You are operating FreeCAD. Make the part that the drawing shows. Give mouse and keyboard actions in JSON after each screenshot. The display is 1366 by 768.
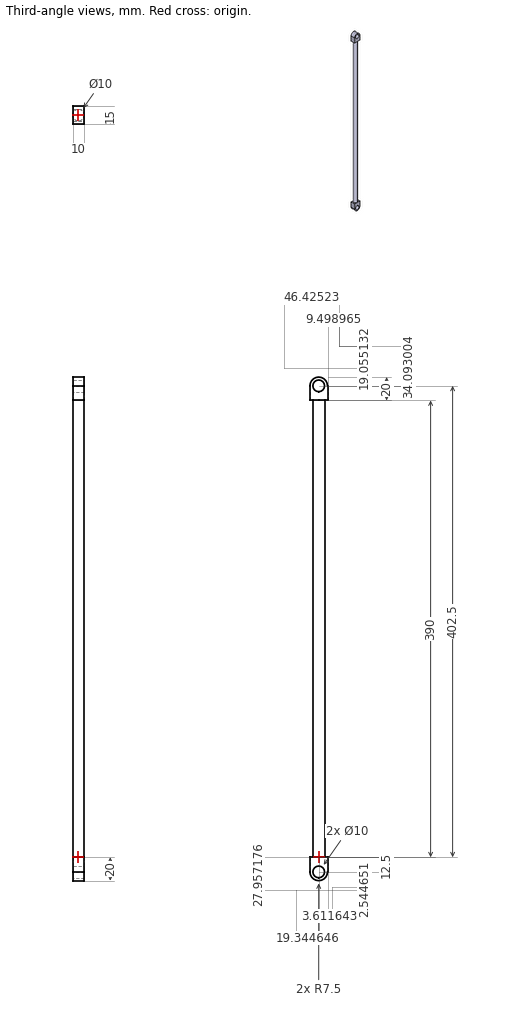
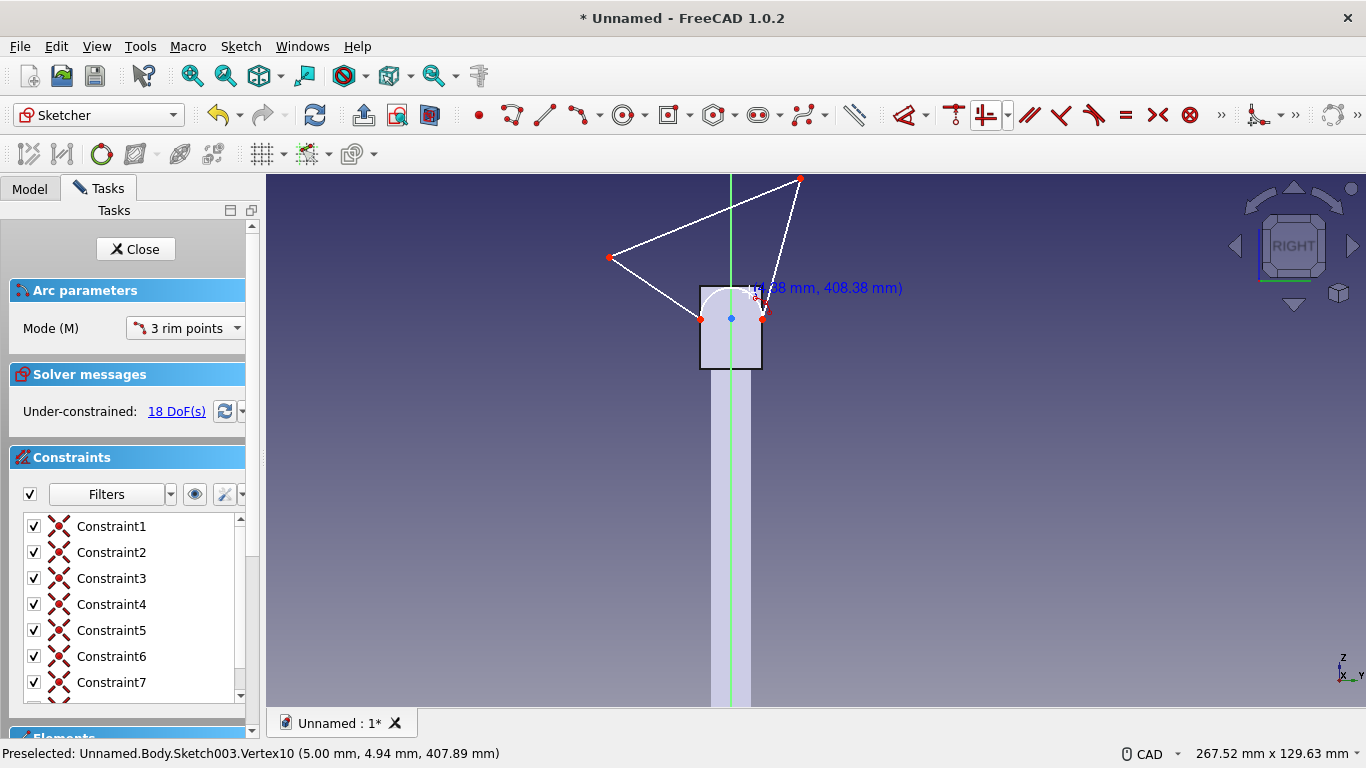
{"action": "left_click", "coordinate": [622, 116]}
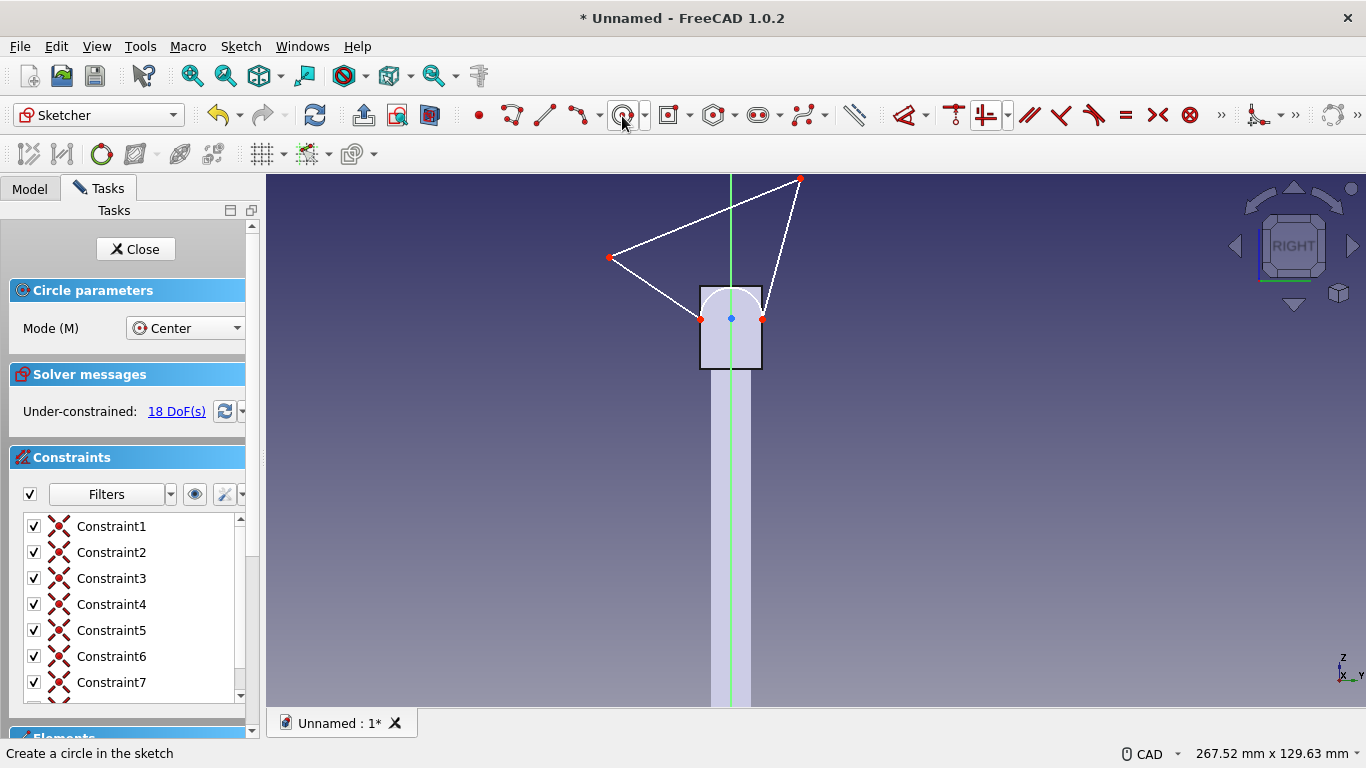
{"action": "scroll", "coordinate": [756, 304], "scroll_direction": "down", "scroll_amount": 9}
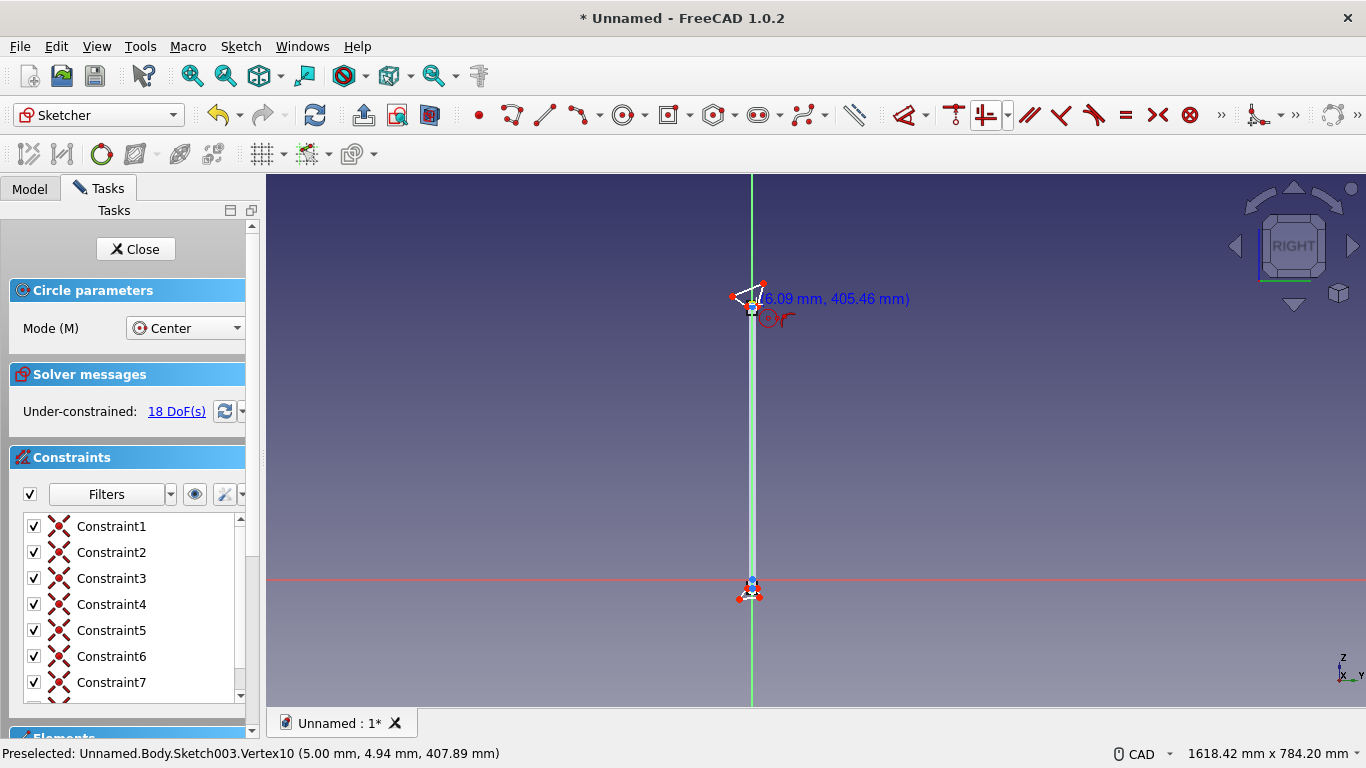
{"action": "scroll", "coordinate": [752, 588], "scroll_direction": "up", "scroll_amount": 10}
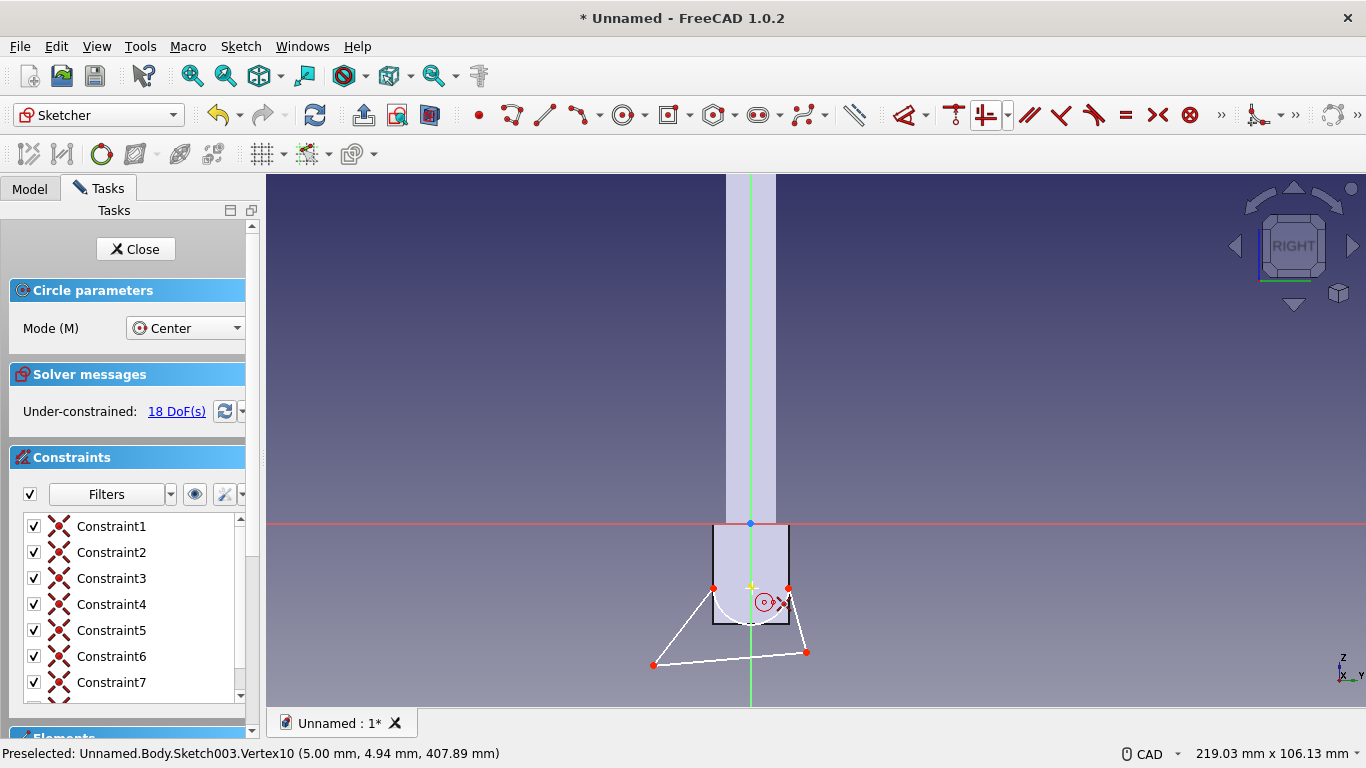
{"action": "left_click", "coordinate": [751, 586]}
{"action": "mouse_move", "coordinate": [769, 569]}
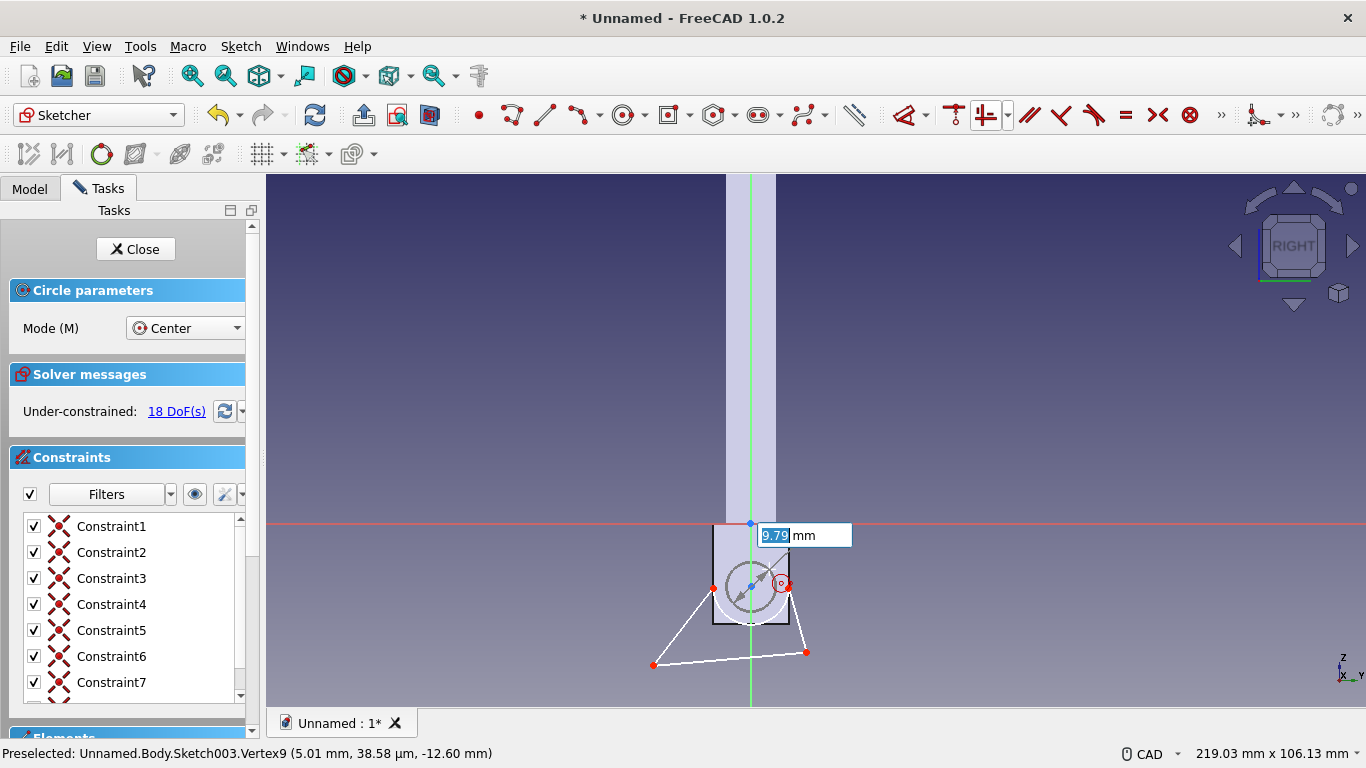
{"action": "type", "text": "10"}
{"action": "key", "text": "Return"}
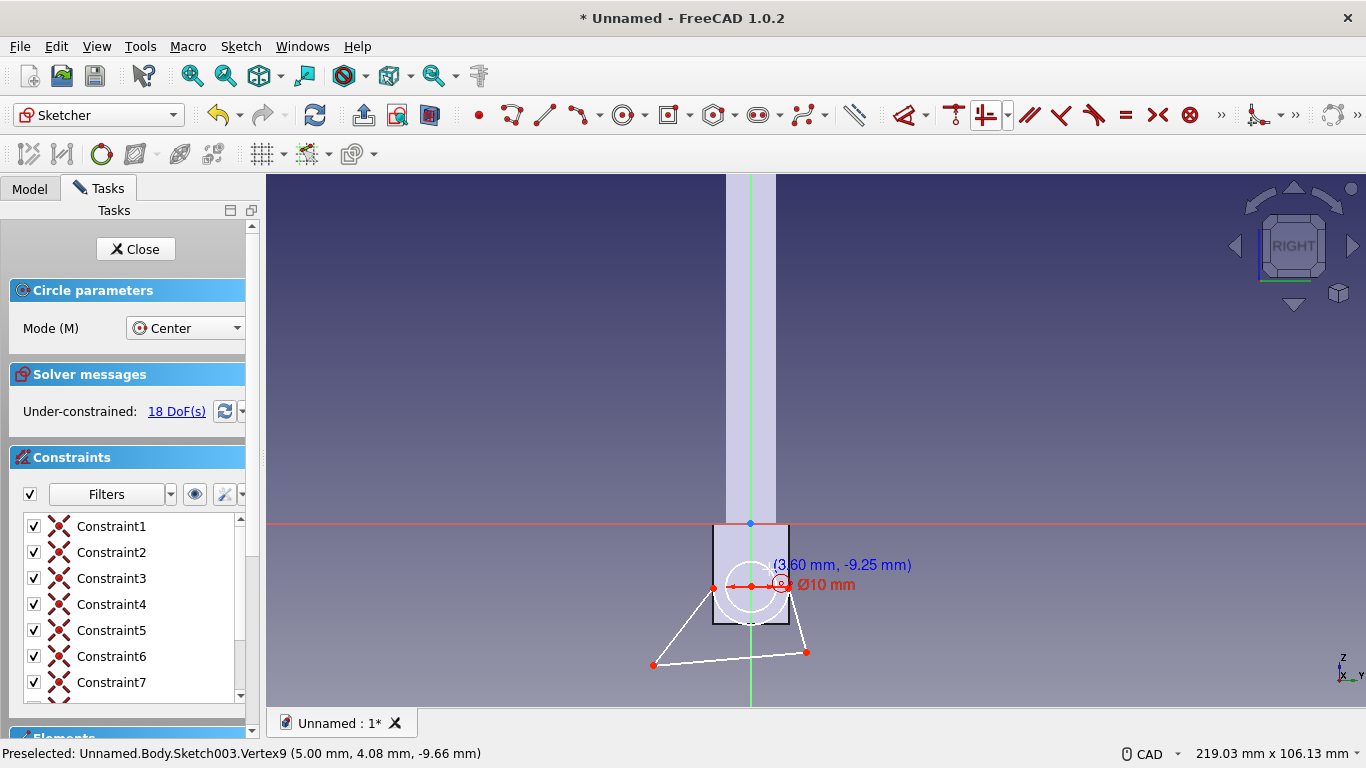
{"action": "scroll", "coordinate": [752, 588], "scroll_direction": "down", "scroll_amount": 10}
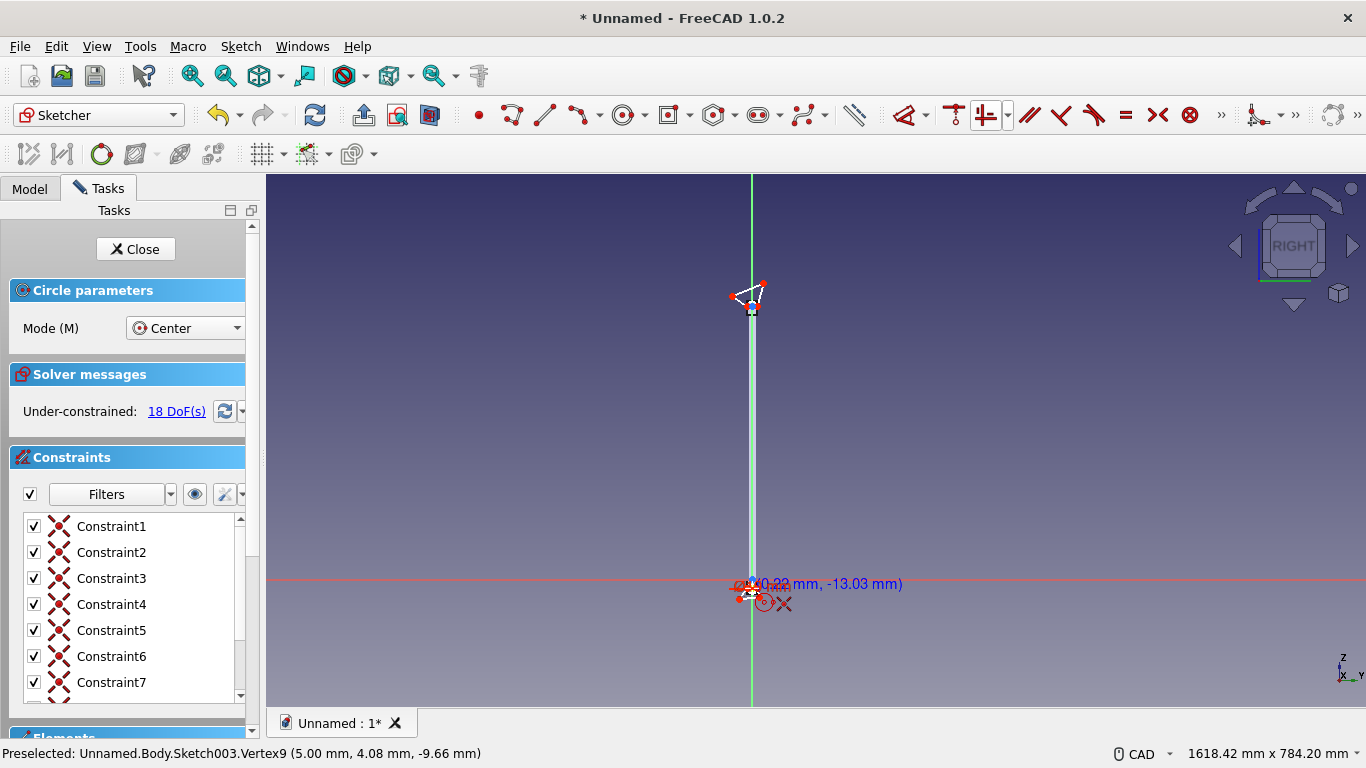
{"action": "scroll", "coordinate": [752, 306], "scroll_direction": "up", "scroll_amount": 10}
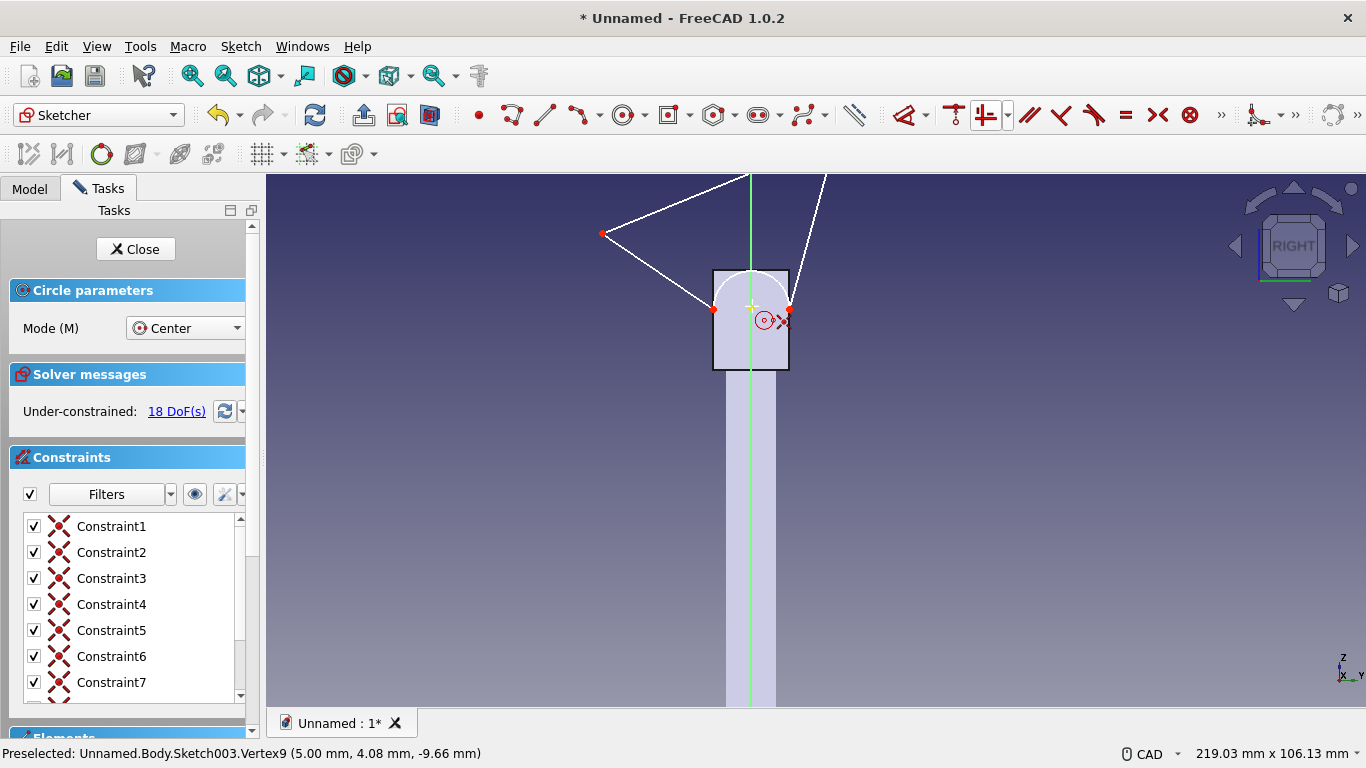
{"action": "left_click", "coordinate": [751, 307]}
{"action": "mouse_move", "coordinate": [769, 325]}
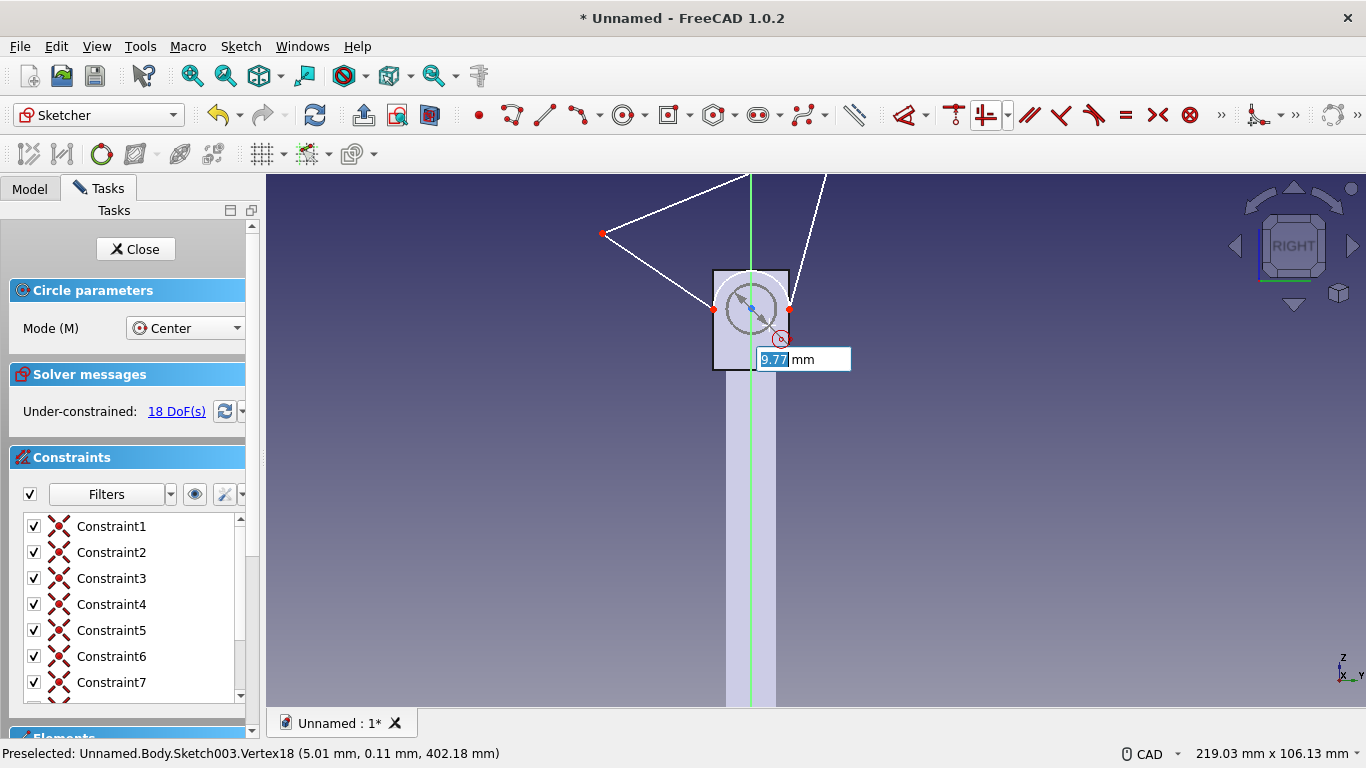
{"action": "type", "text": "10"}
{"action": "key", "text": "Return"}
{"action": "key", "text": "Escape"}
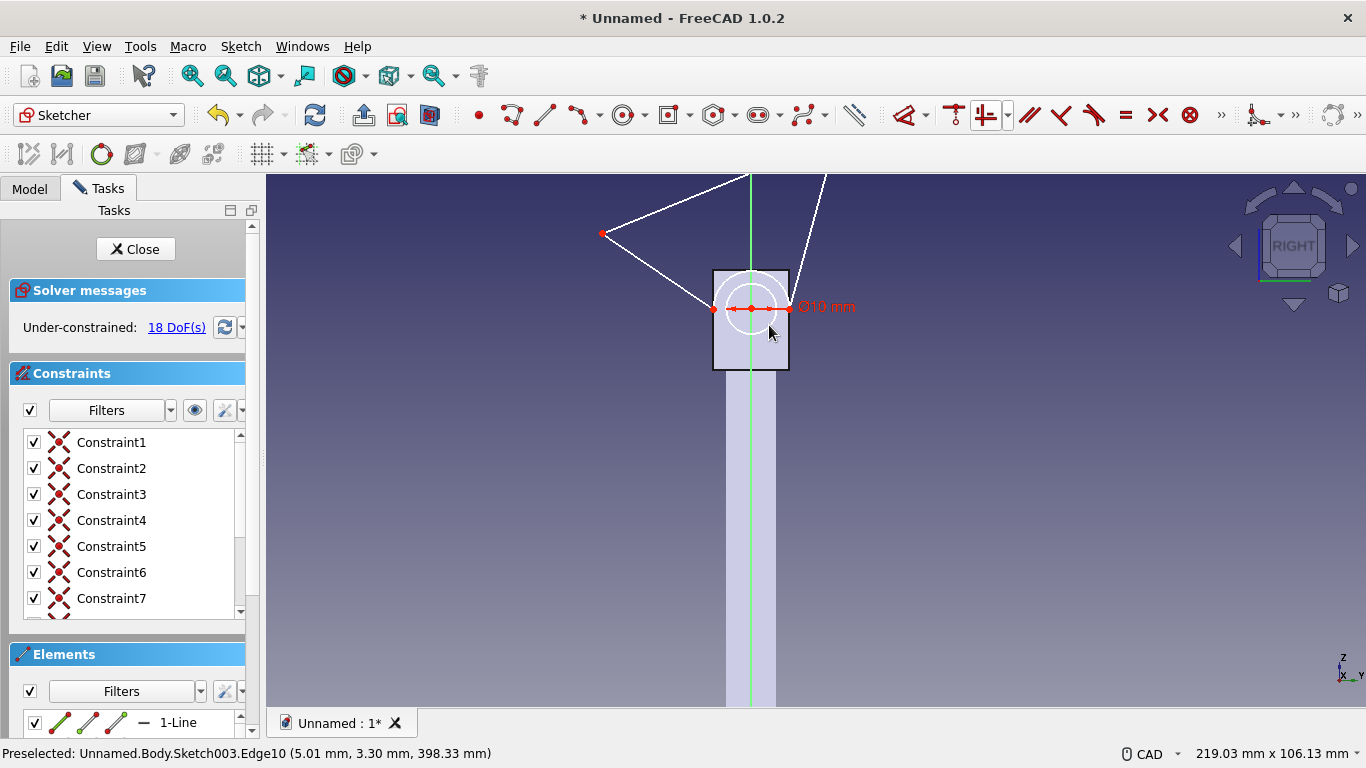
{"action": "scroll", "coordinate": [752, 306], "scroll_direction": "down", "scroll_amount": 10}